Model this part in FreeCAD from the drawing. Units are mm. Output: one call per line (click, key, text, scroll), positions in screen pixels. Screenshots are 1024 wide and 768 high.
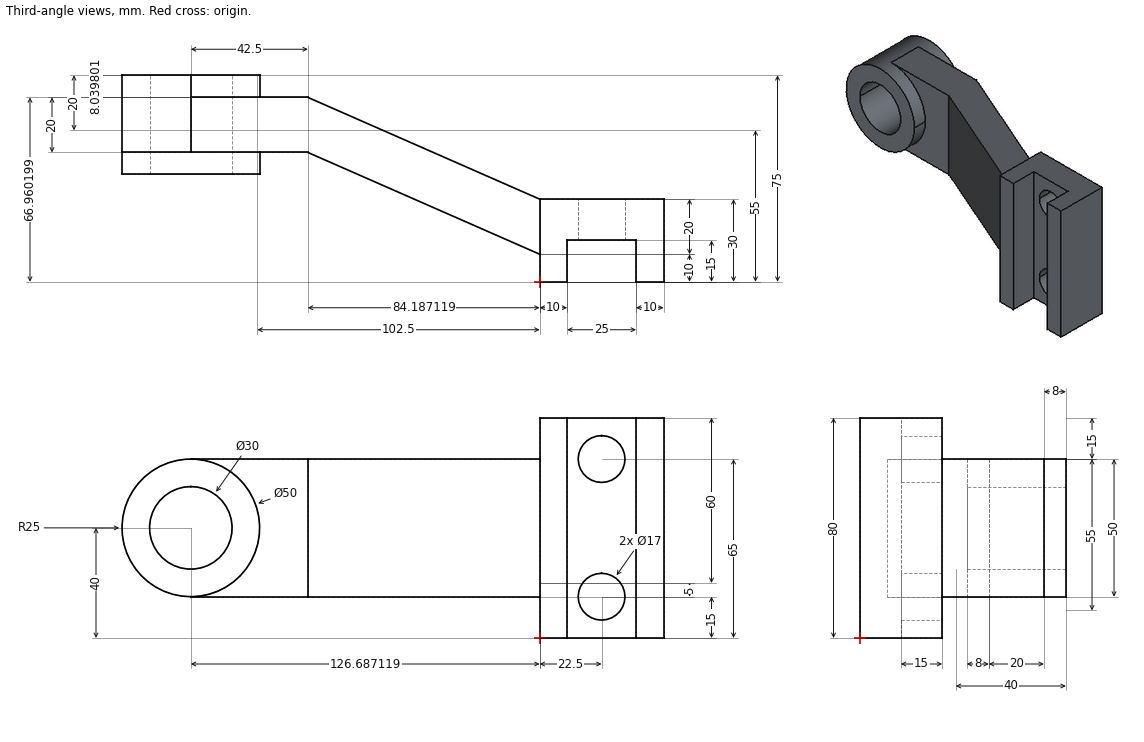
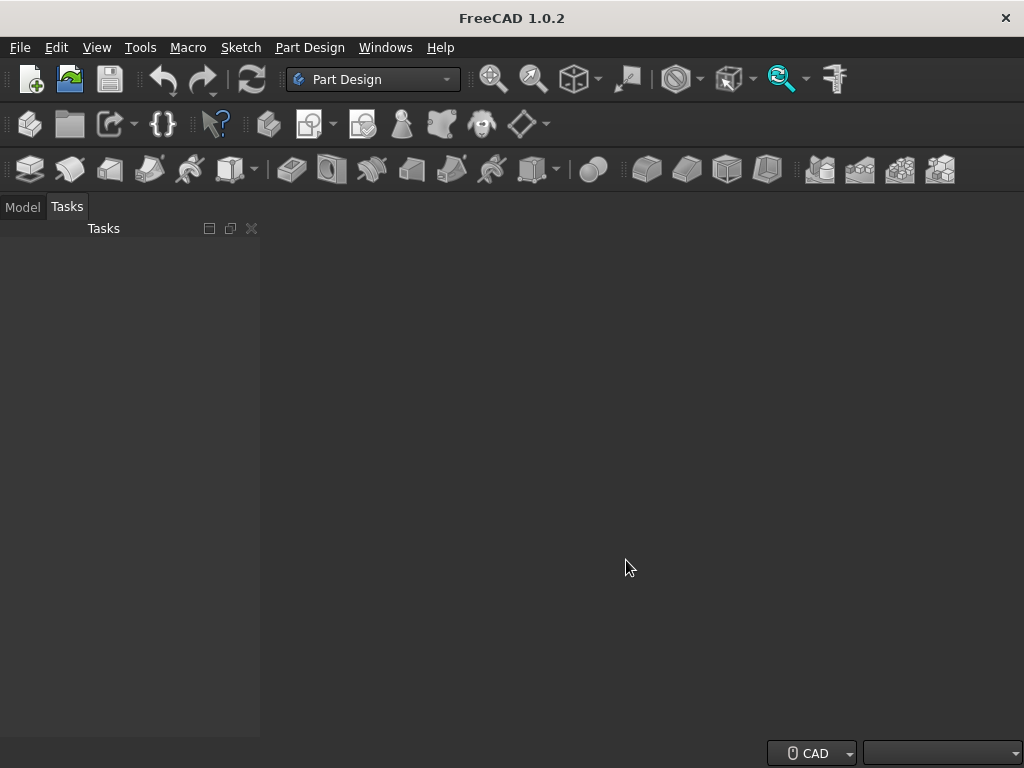
key(ctrl+n)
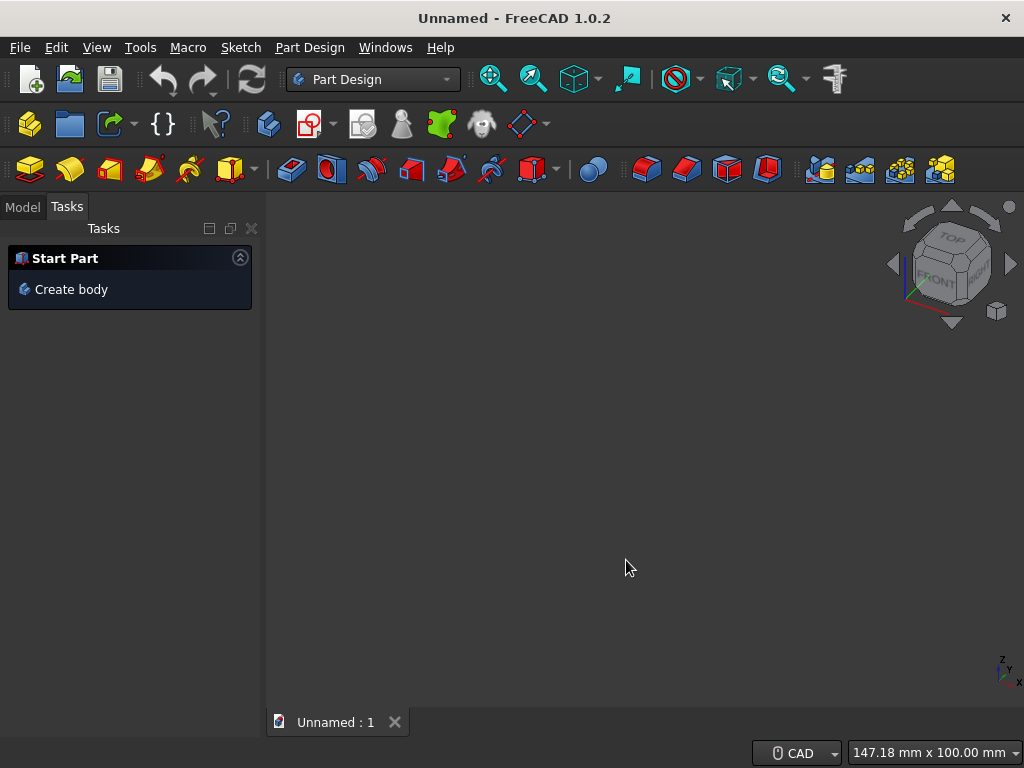
click(310, 124)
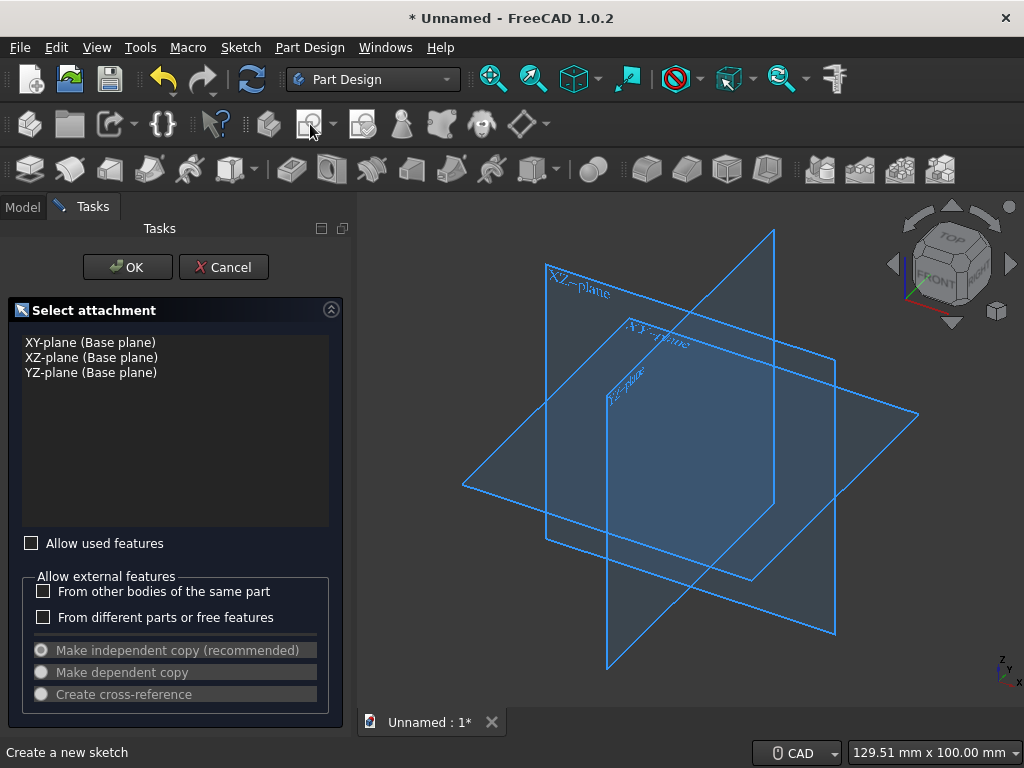
click(82, 342)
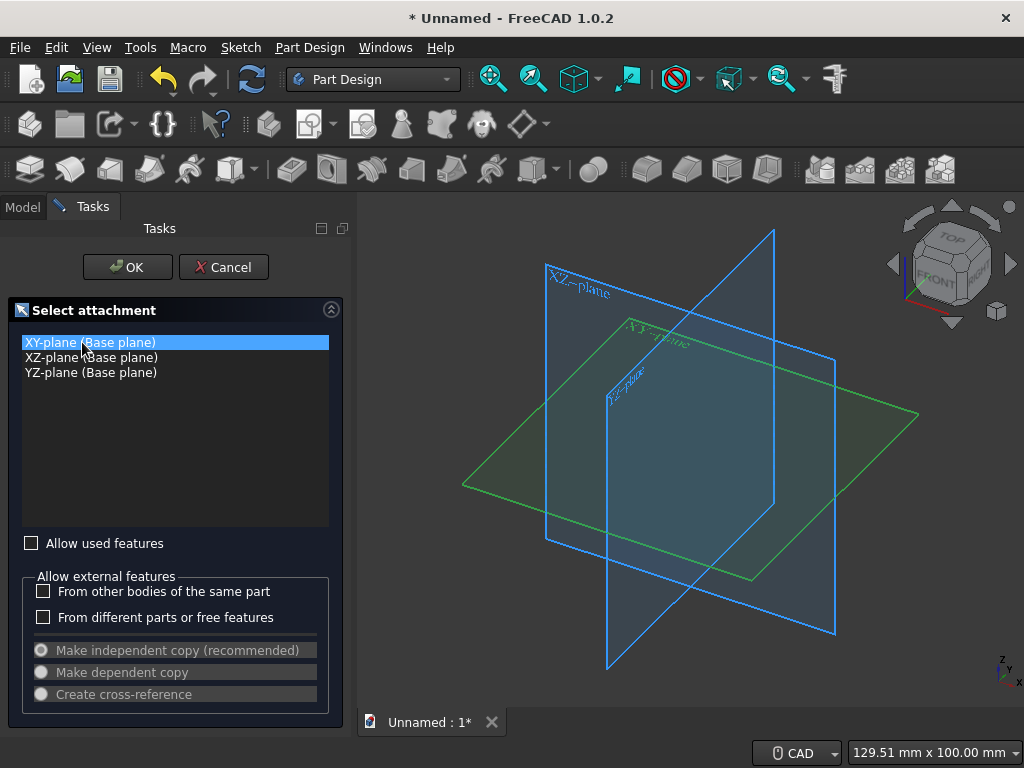
click(128, 267)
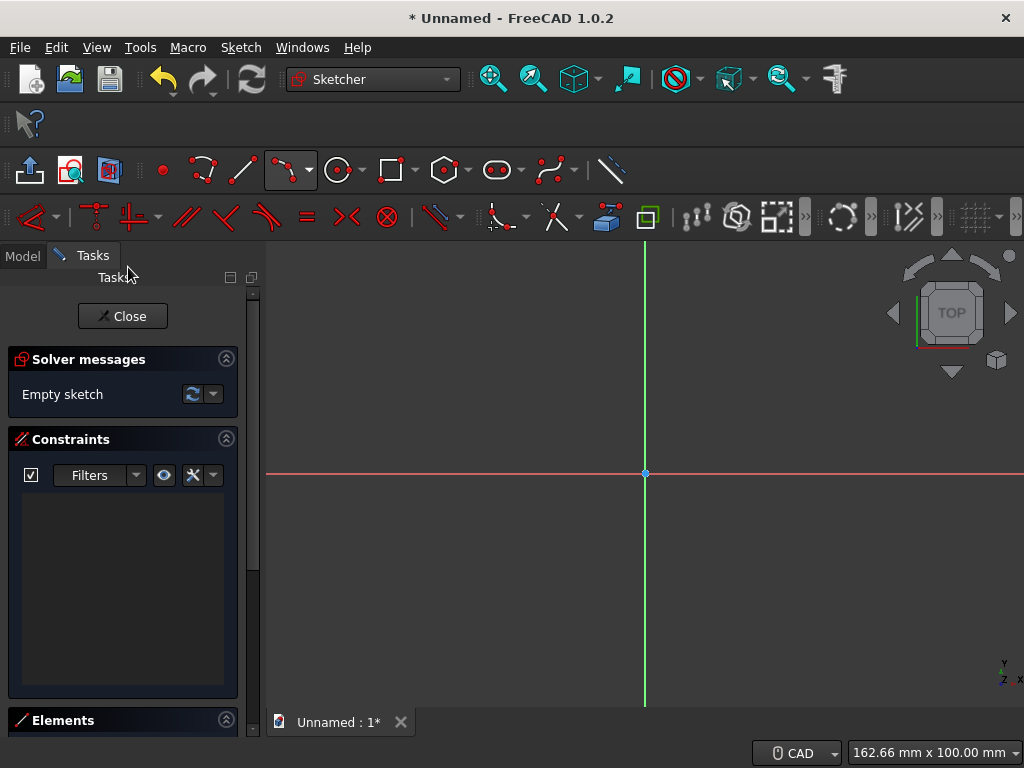
scroll(576, 474, down, 5)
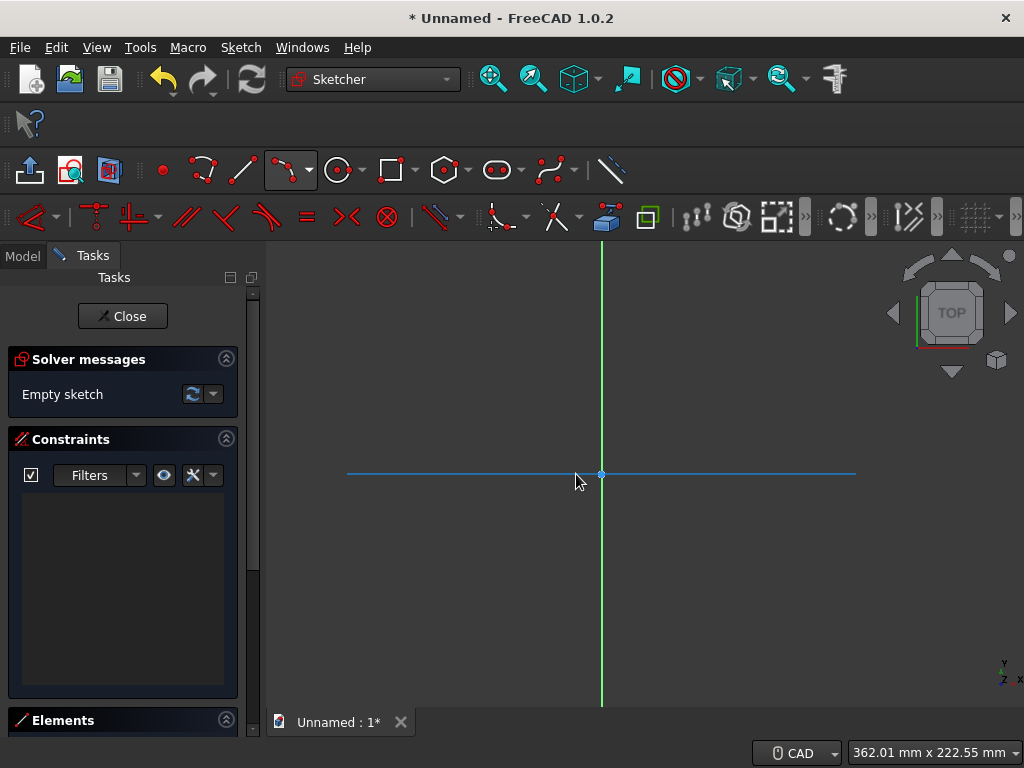
scroll(656, 442, up, 8)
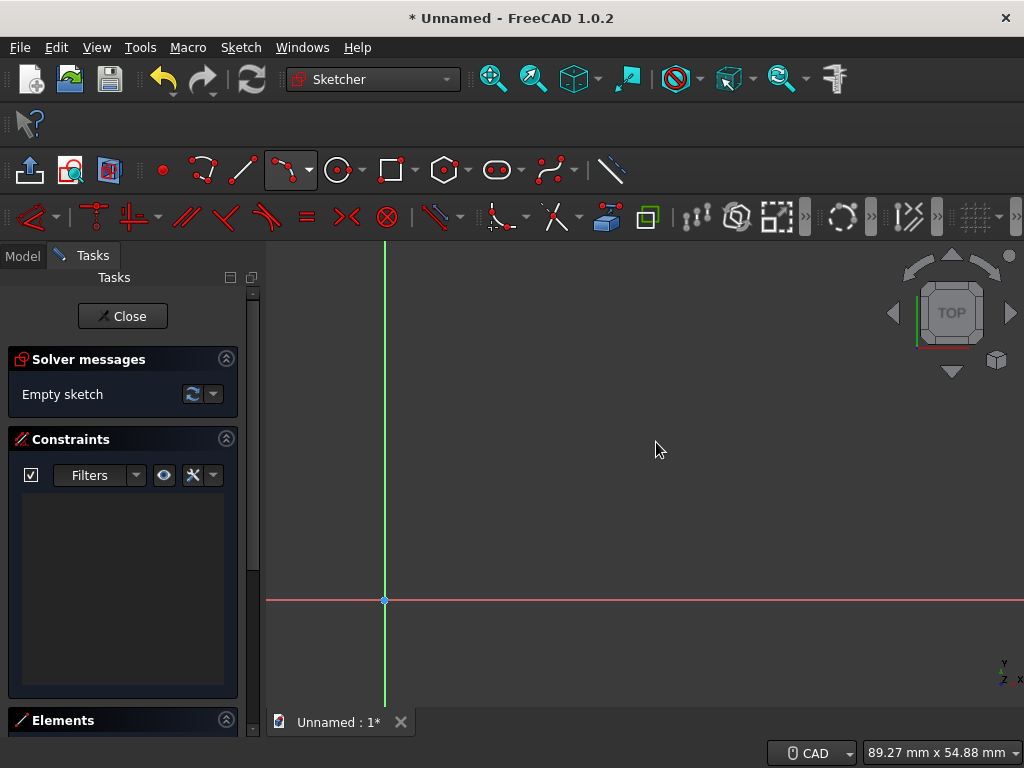
click(204, 170)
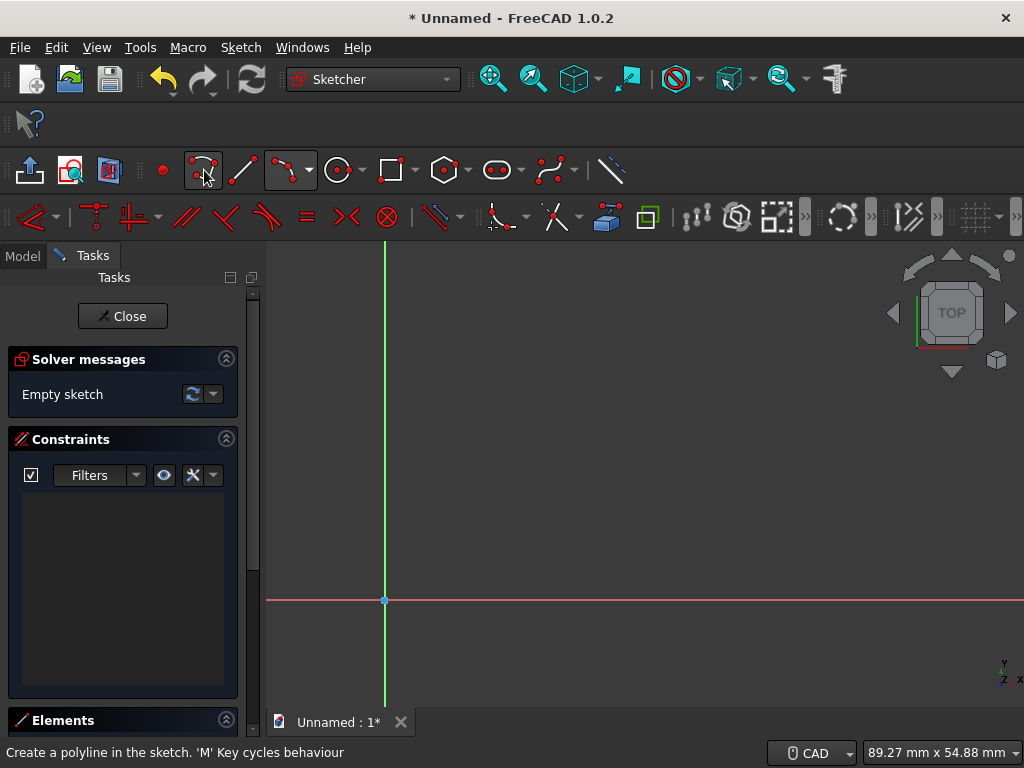
click(385, 600)
click(470, 591)
click(470, 473)
click(682, 473)
click(682, 600)
click(767, 591)
click(767, 346)
click(394, 346)
click(385, 600)
key(Escape)
key(Escape)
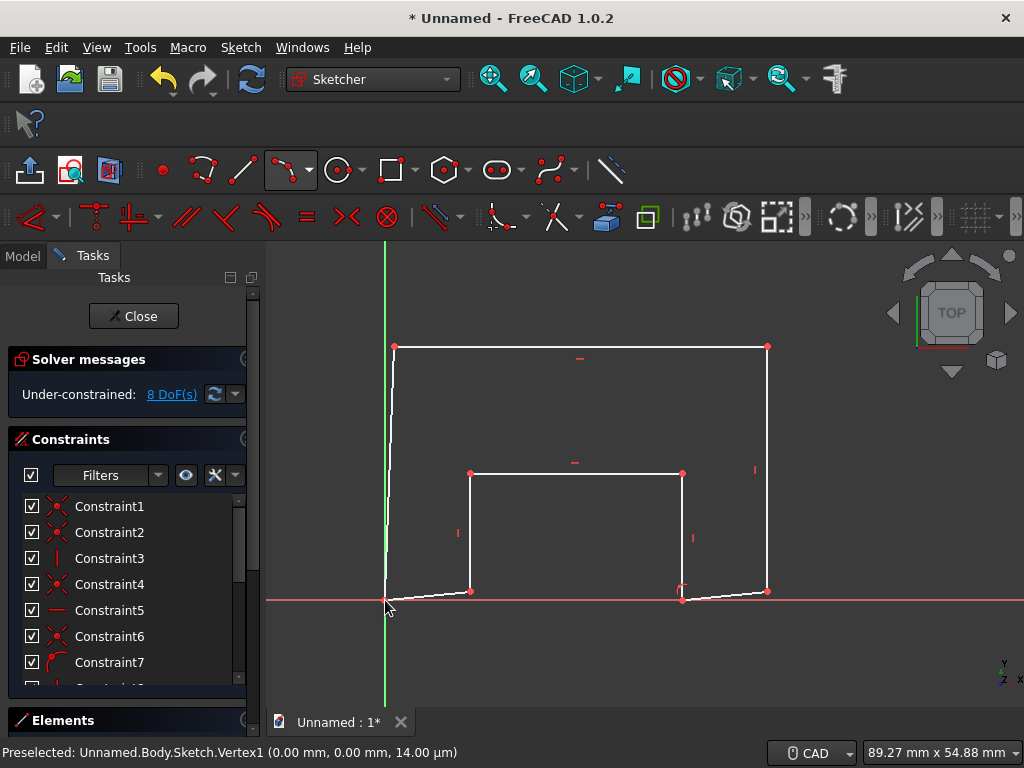
click(410, 598)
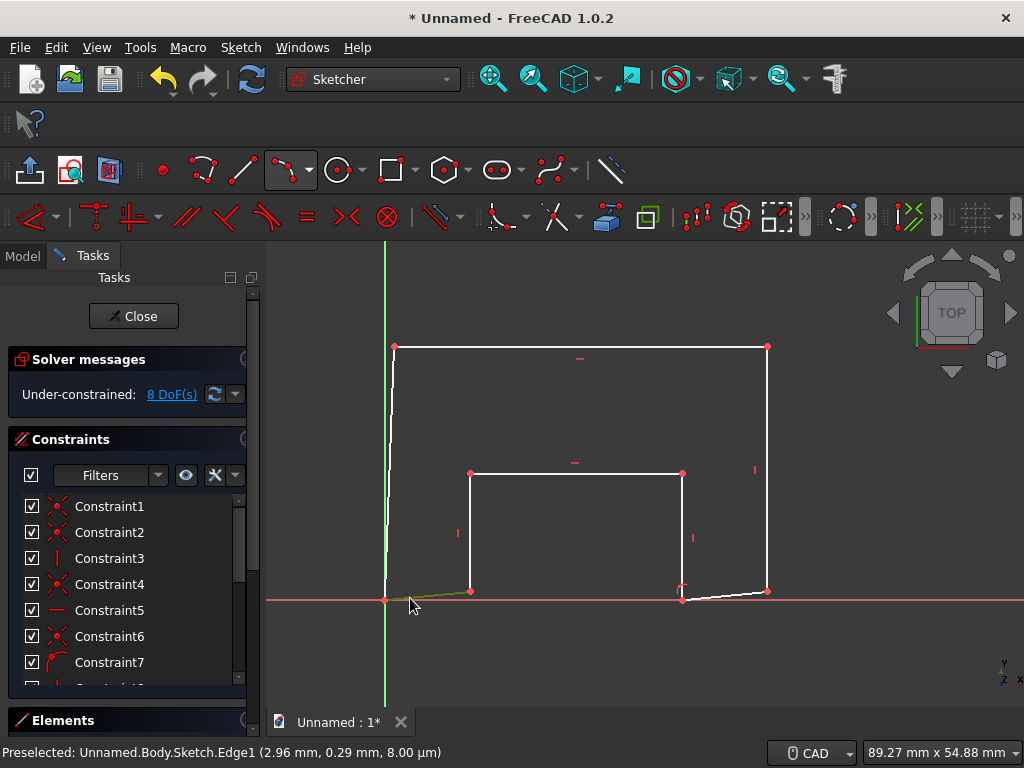
key(h)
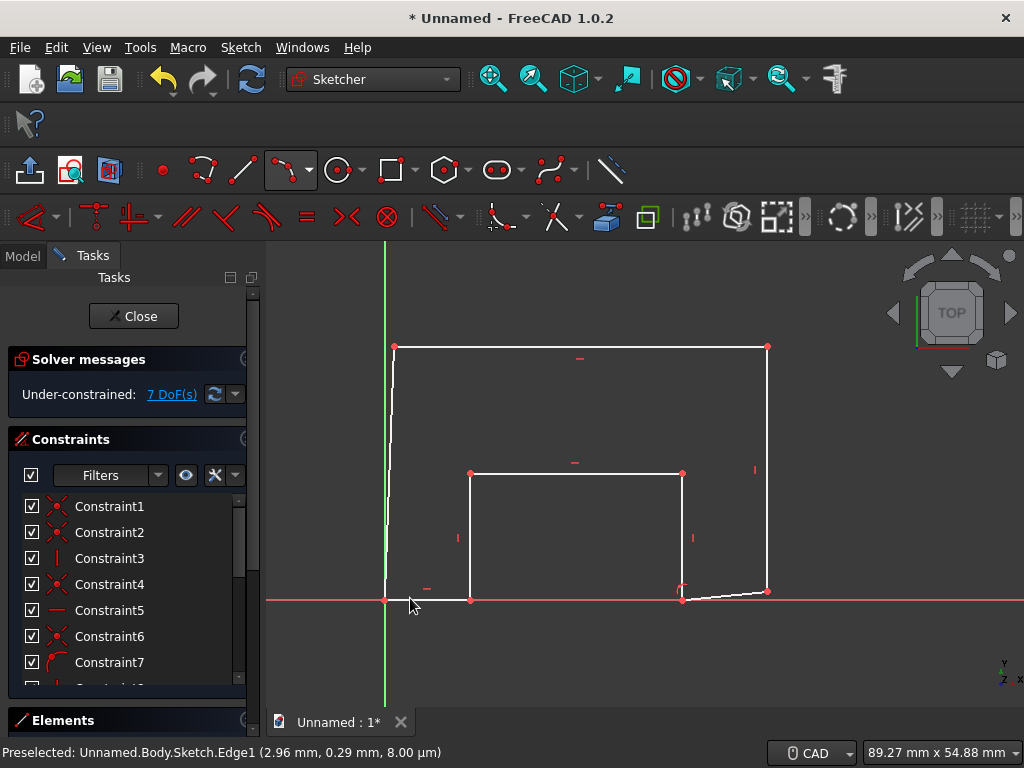
click(707, 598)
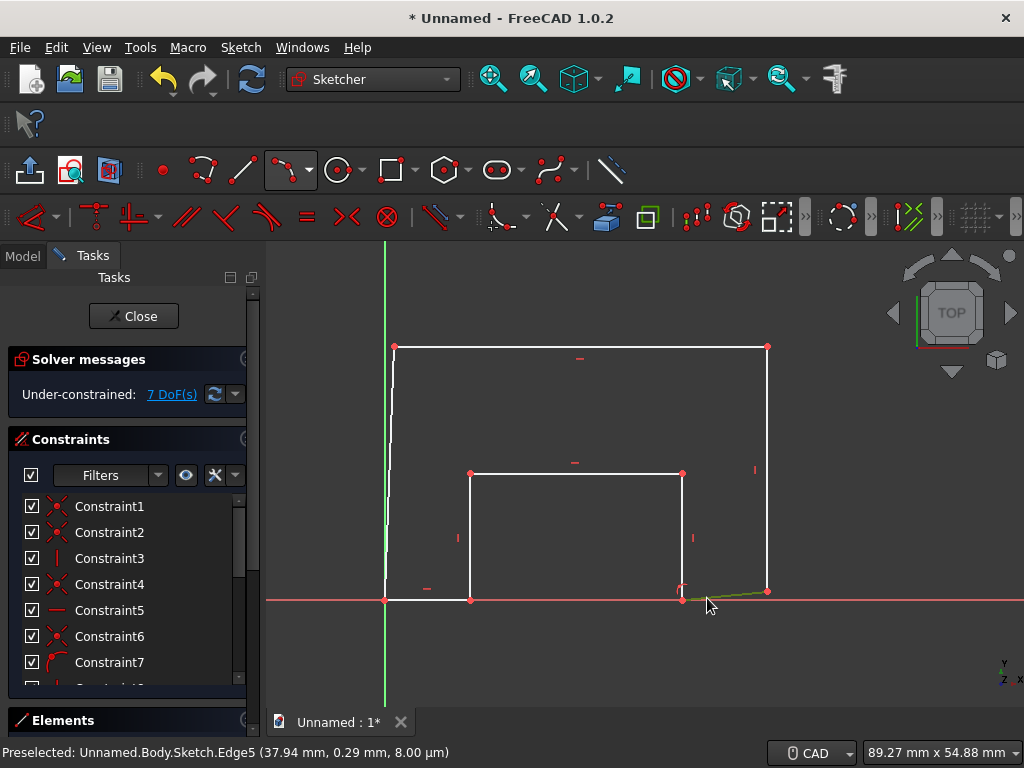
key(h)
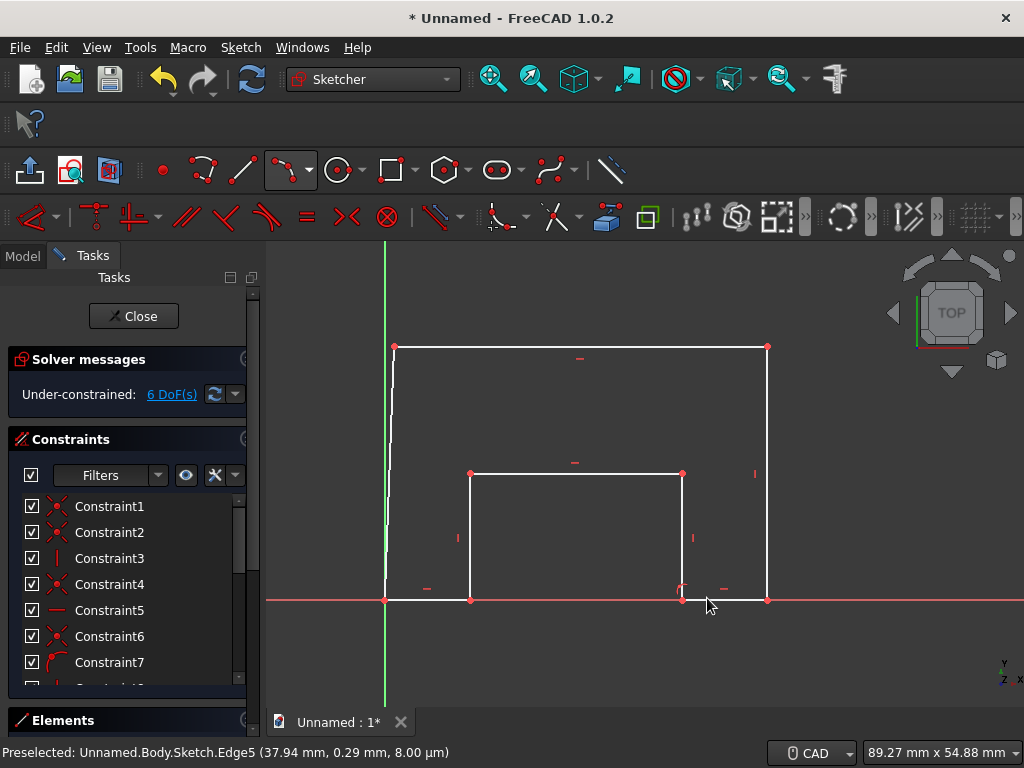
click(388, 524)